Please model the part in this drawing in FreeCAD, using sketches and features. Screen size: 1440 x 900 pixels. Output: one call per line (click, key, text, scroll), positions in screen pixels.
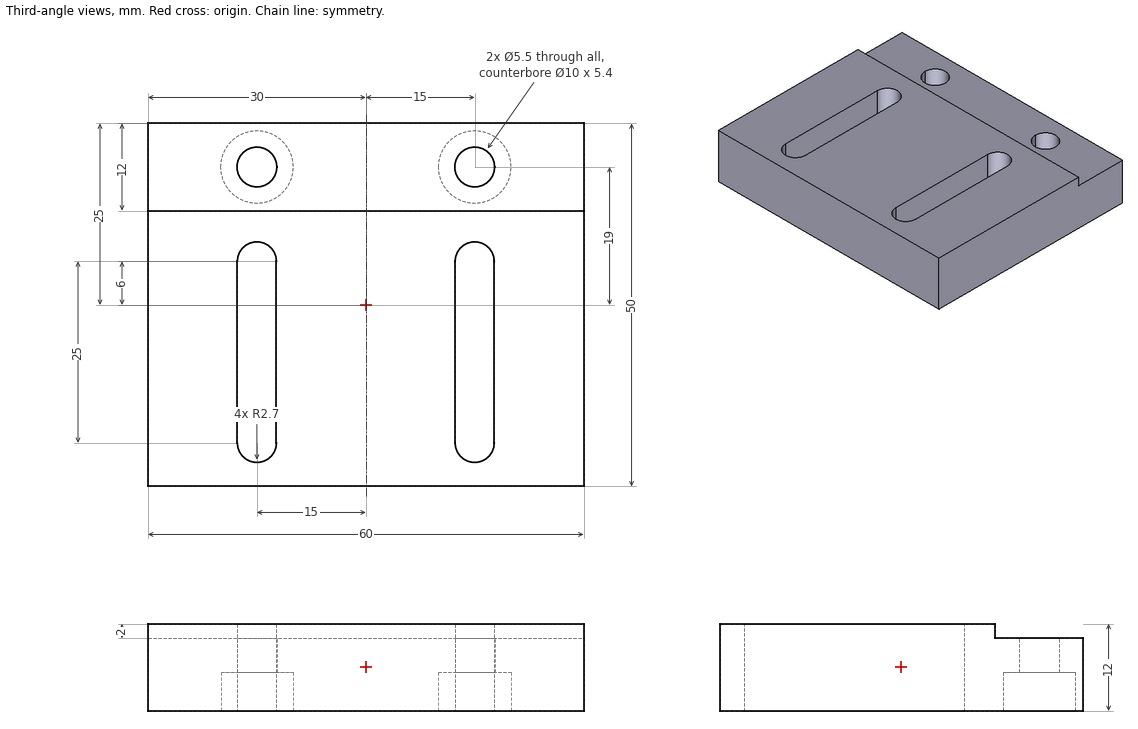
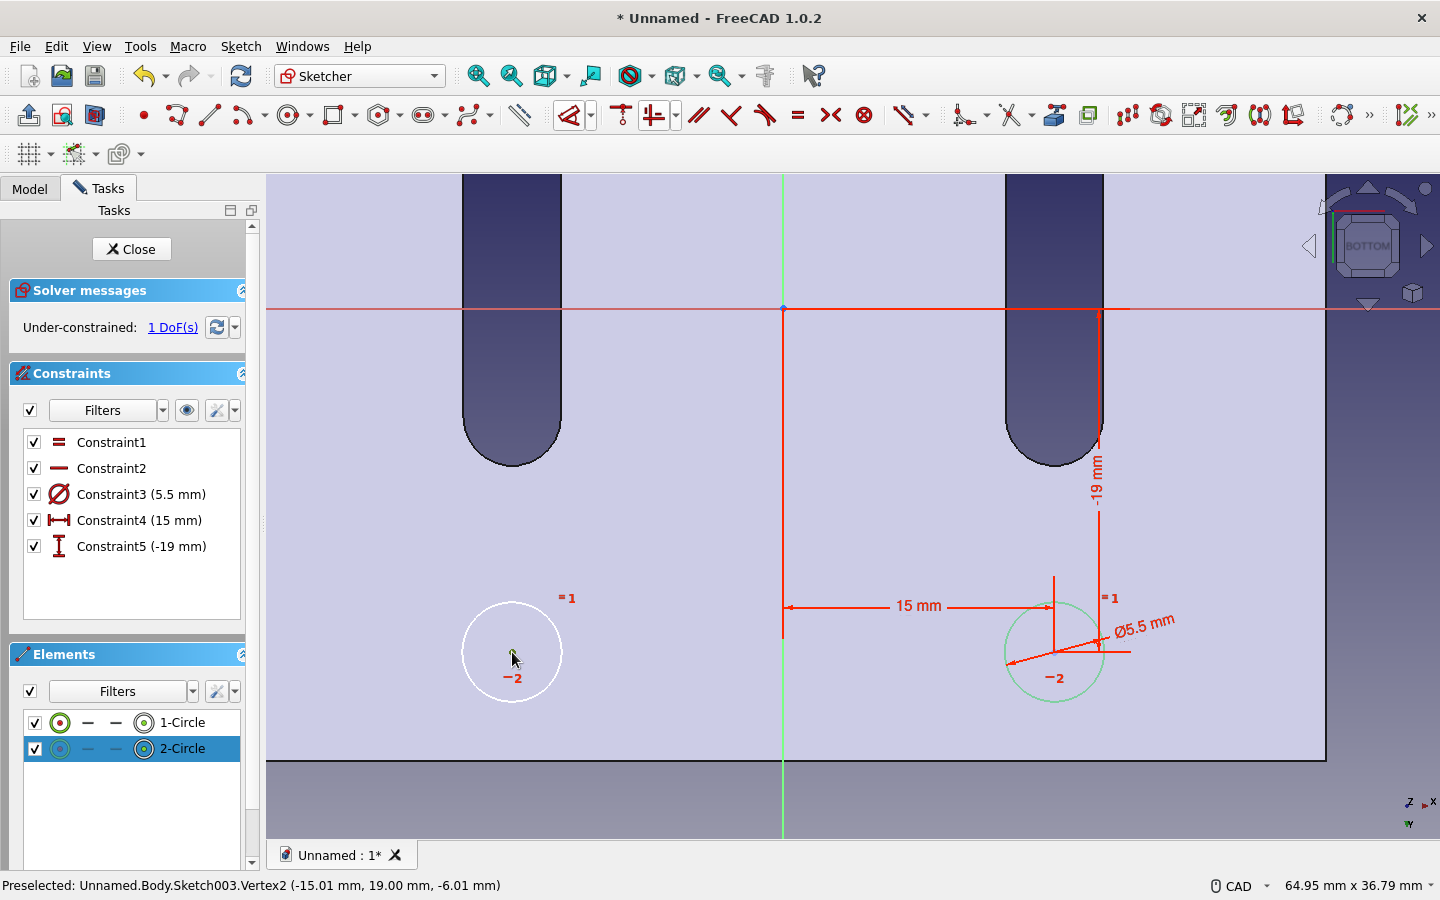
key(l)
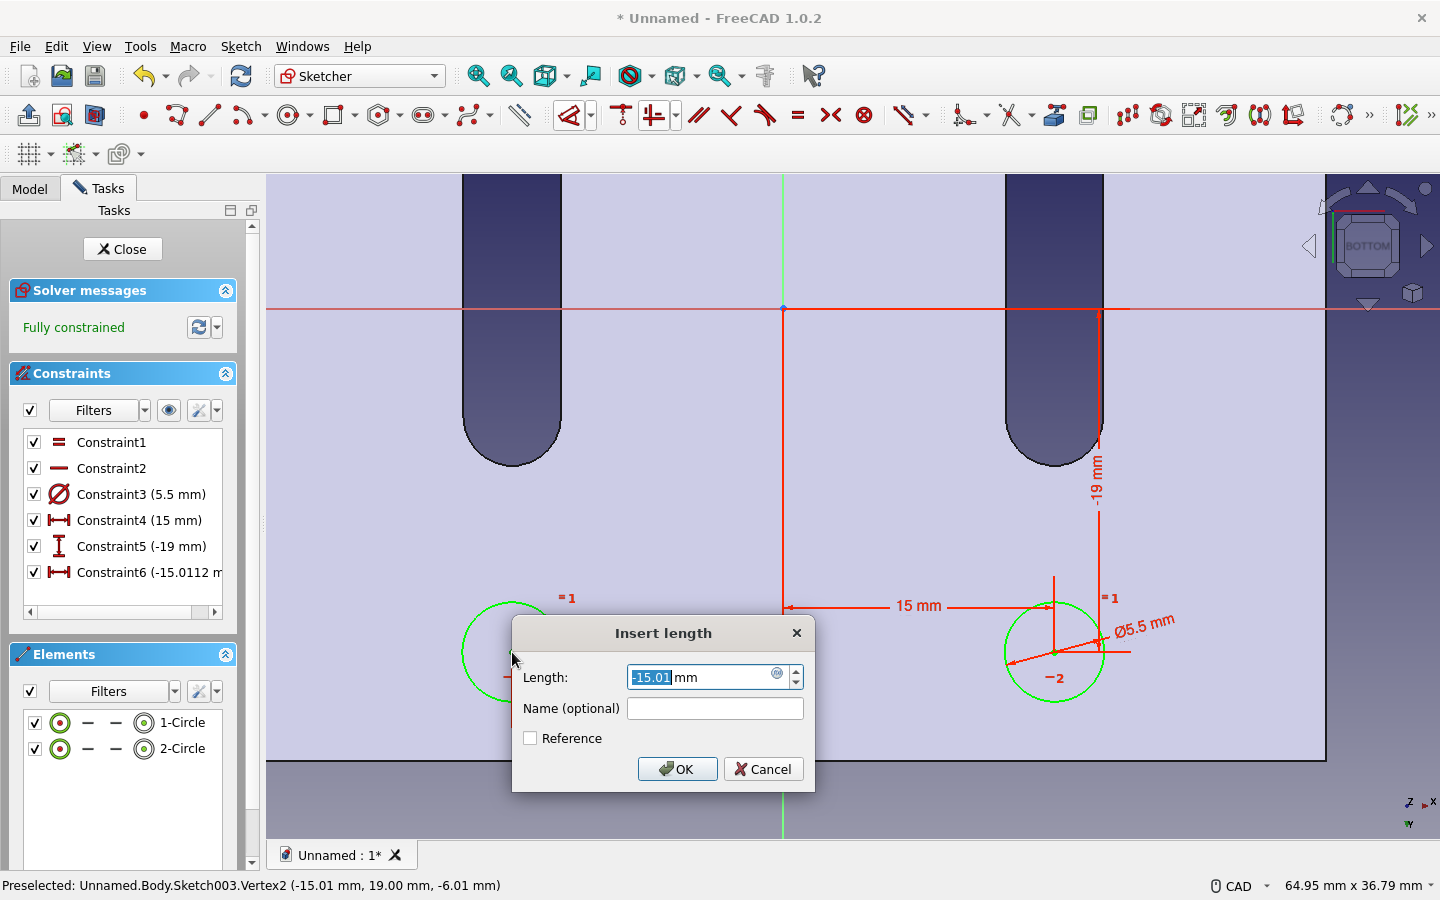
text(-15)
key(Return)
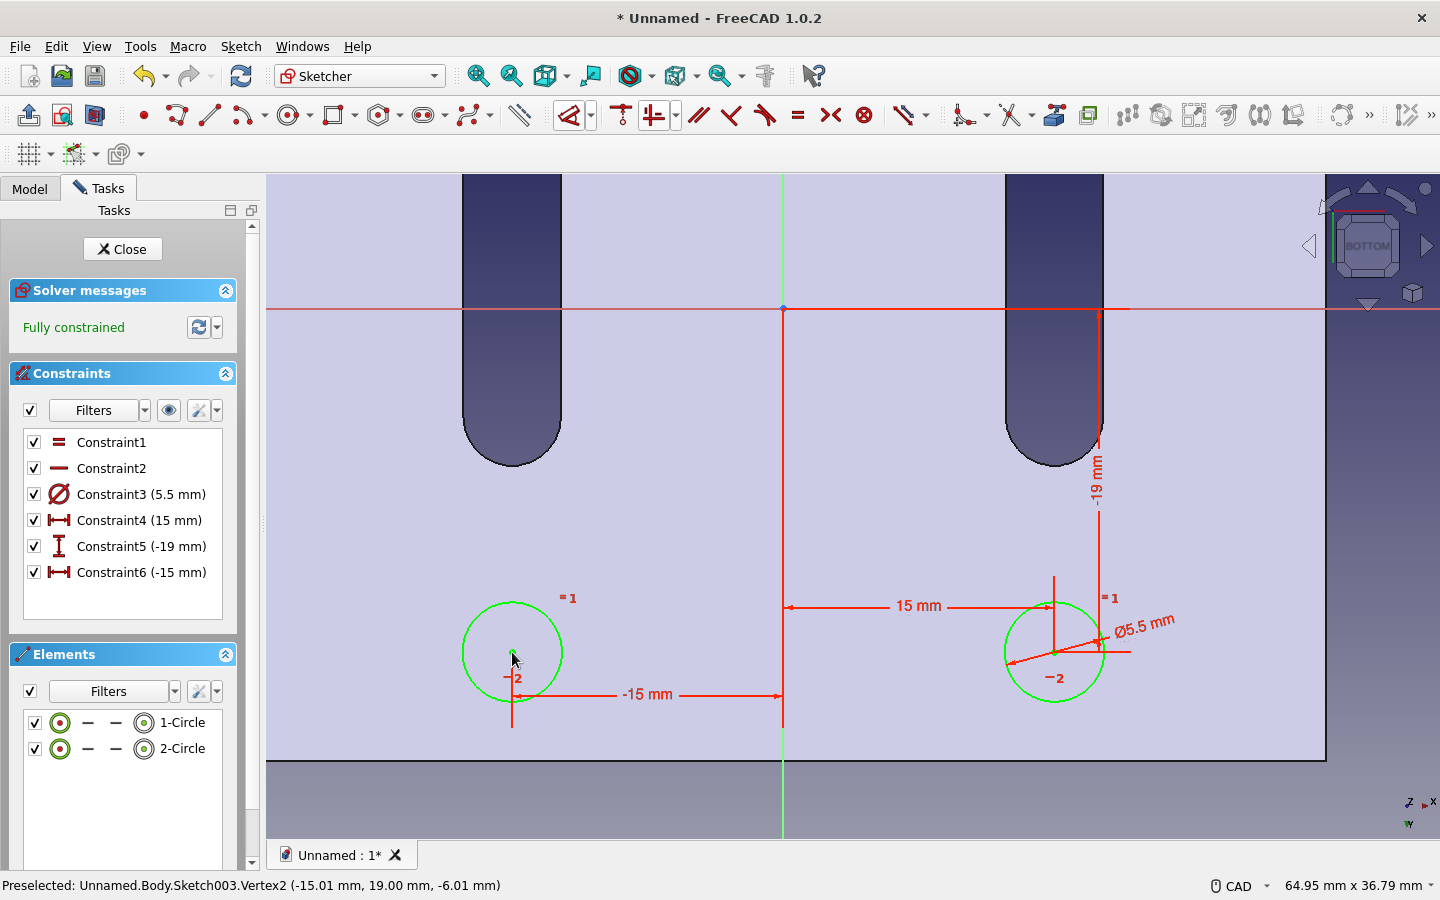
click(123, 249)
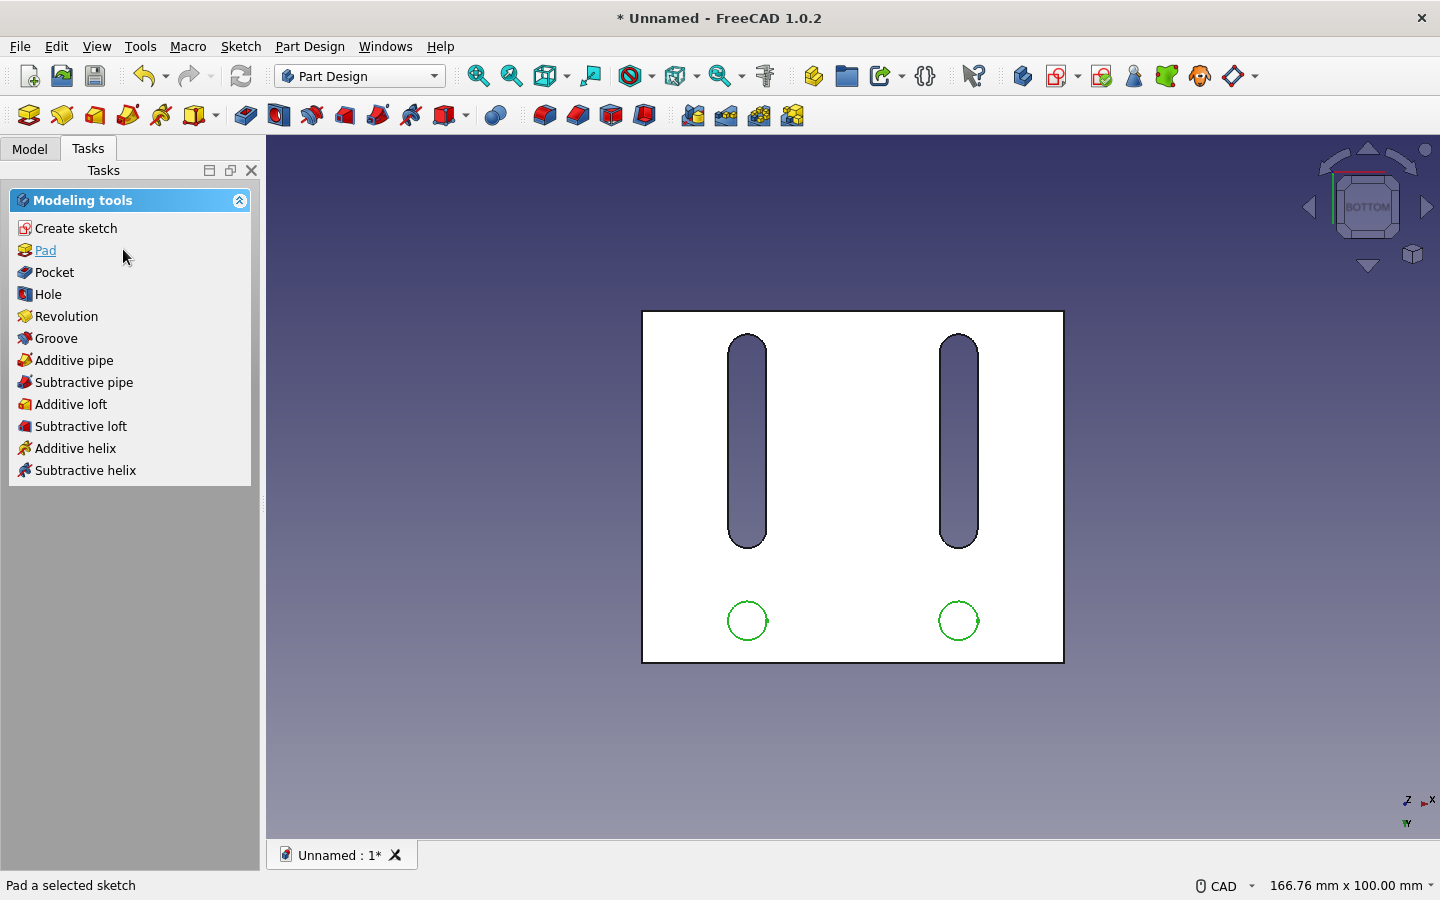
click(279, 116)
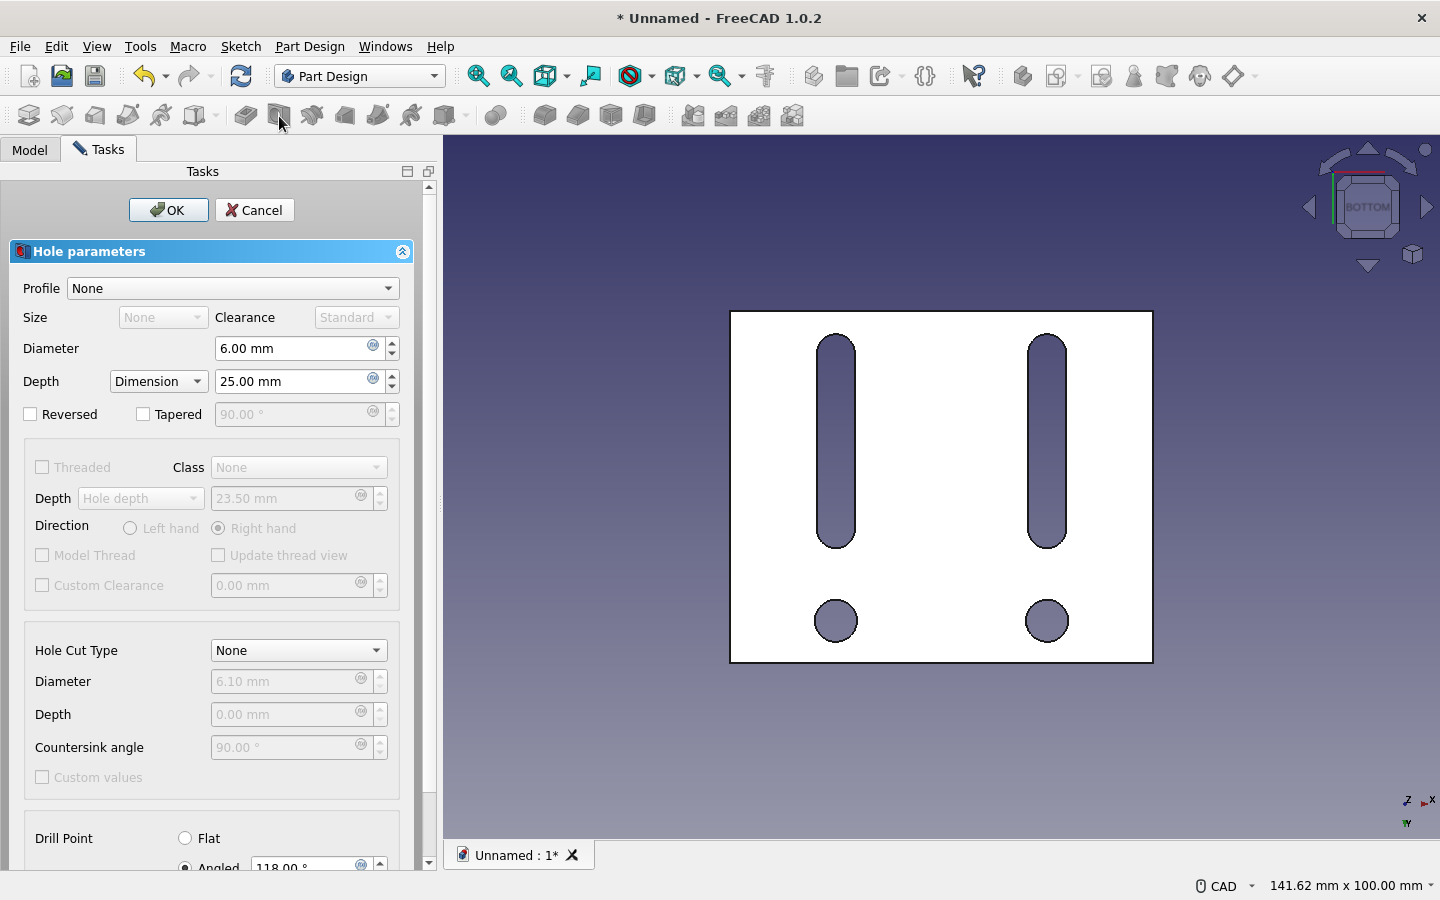
triple_click(300, 348)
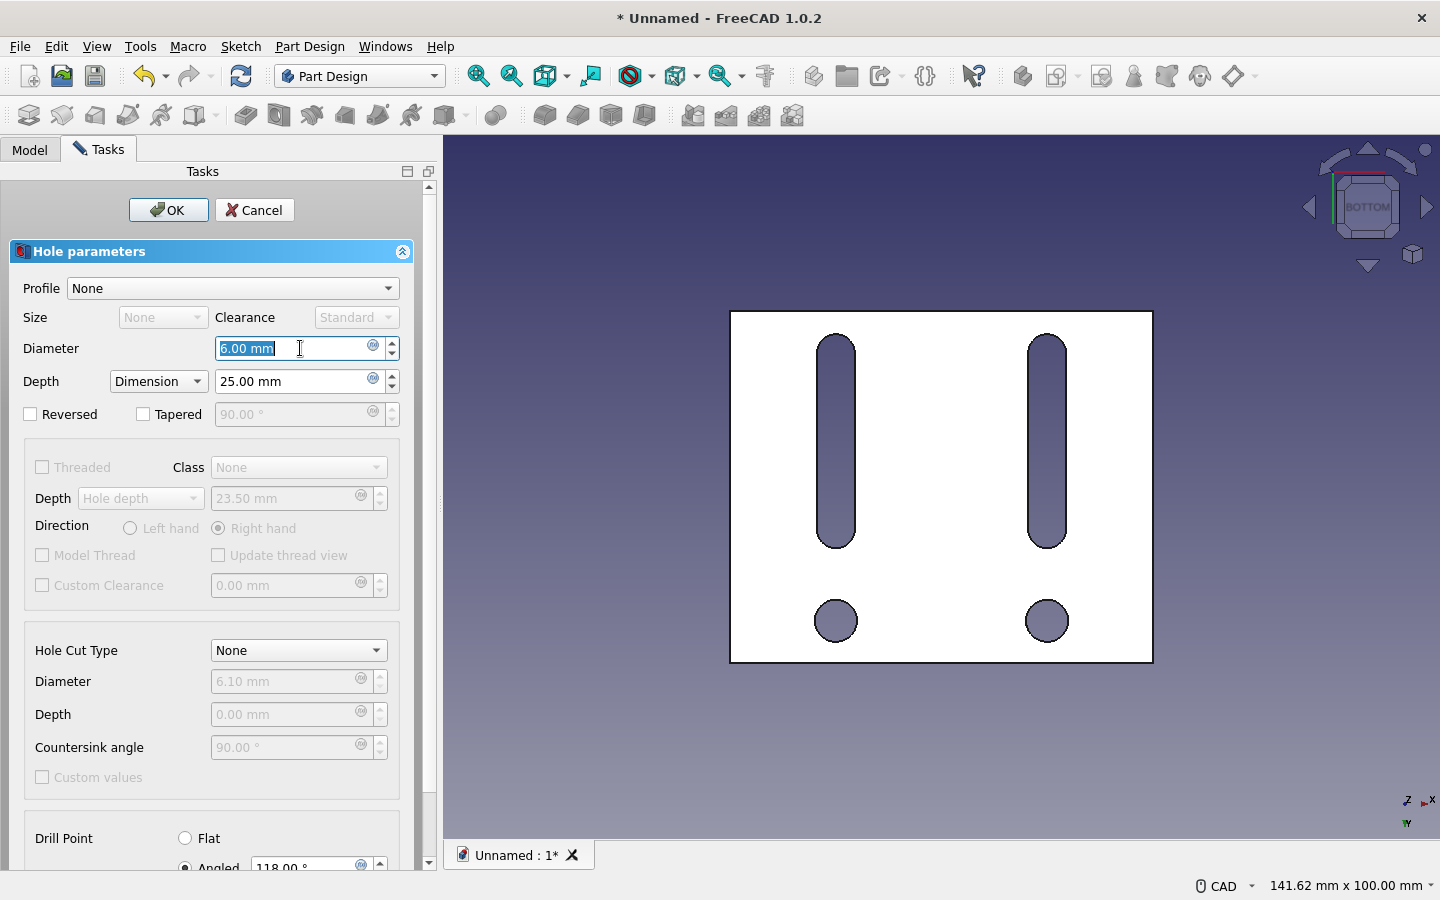
text(5.5)
key(Tab)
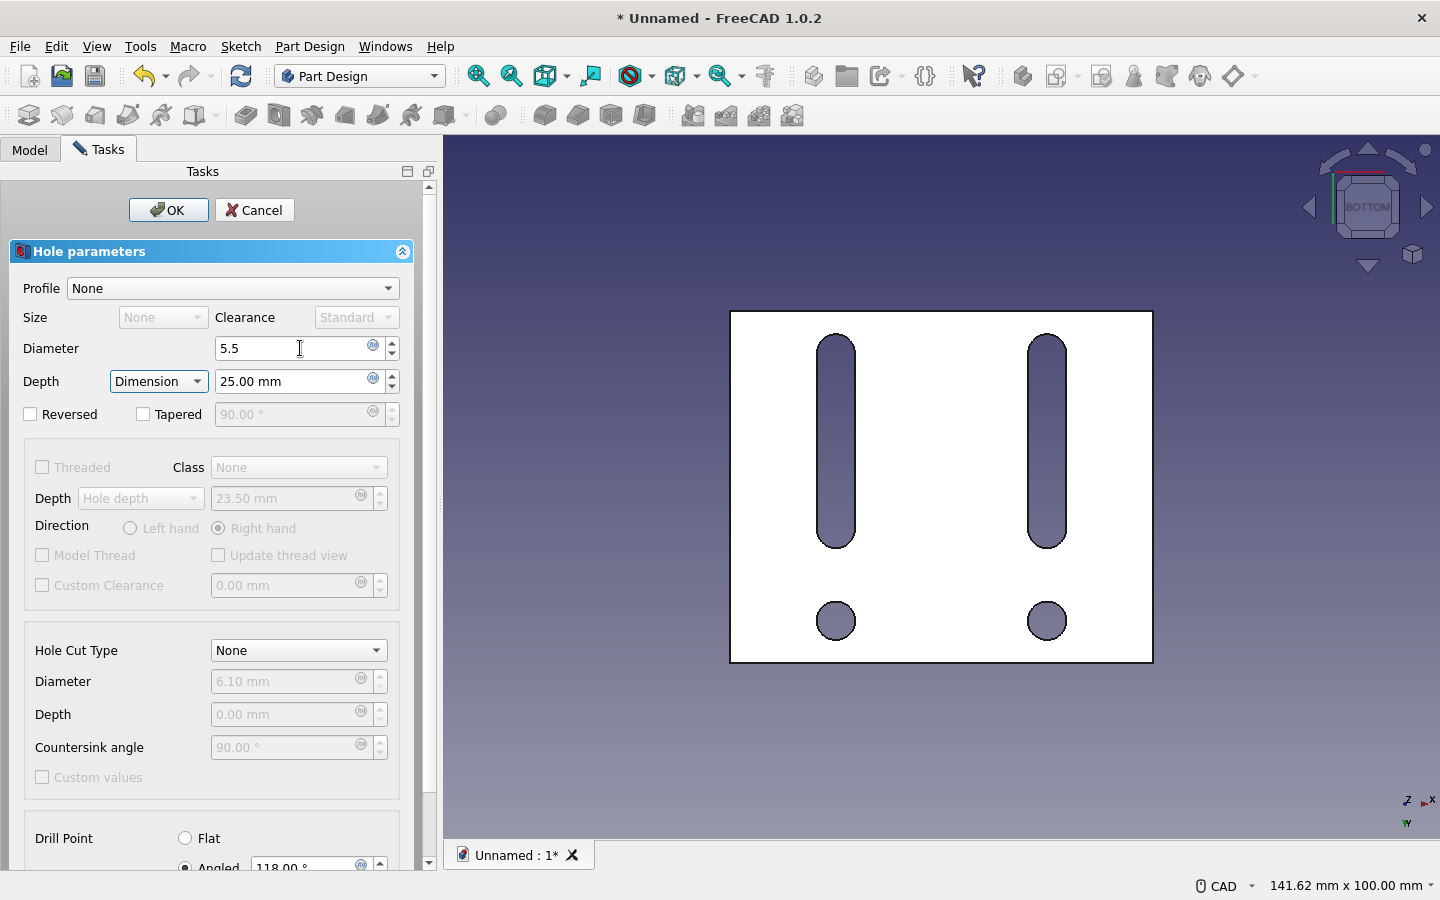
click(160, 382)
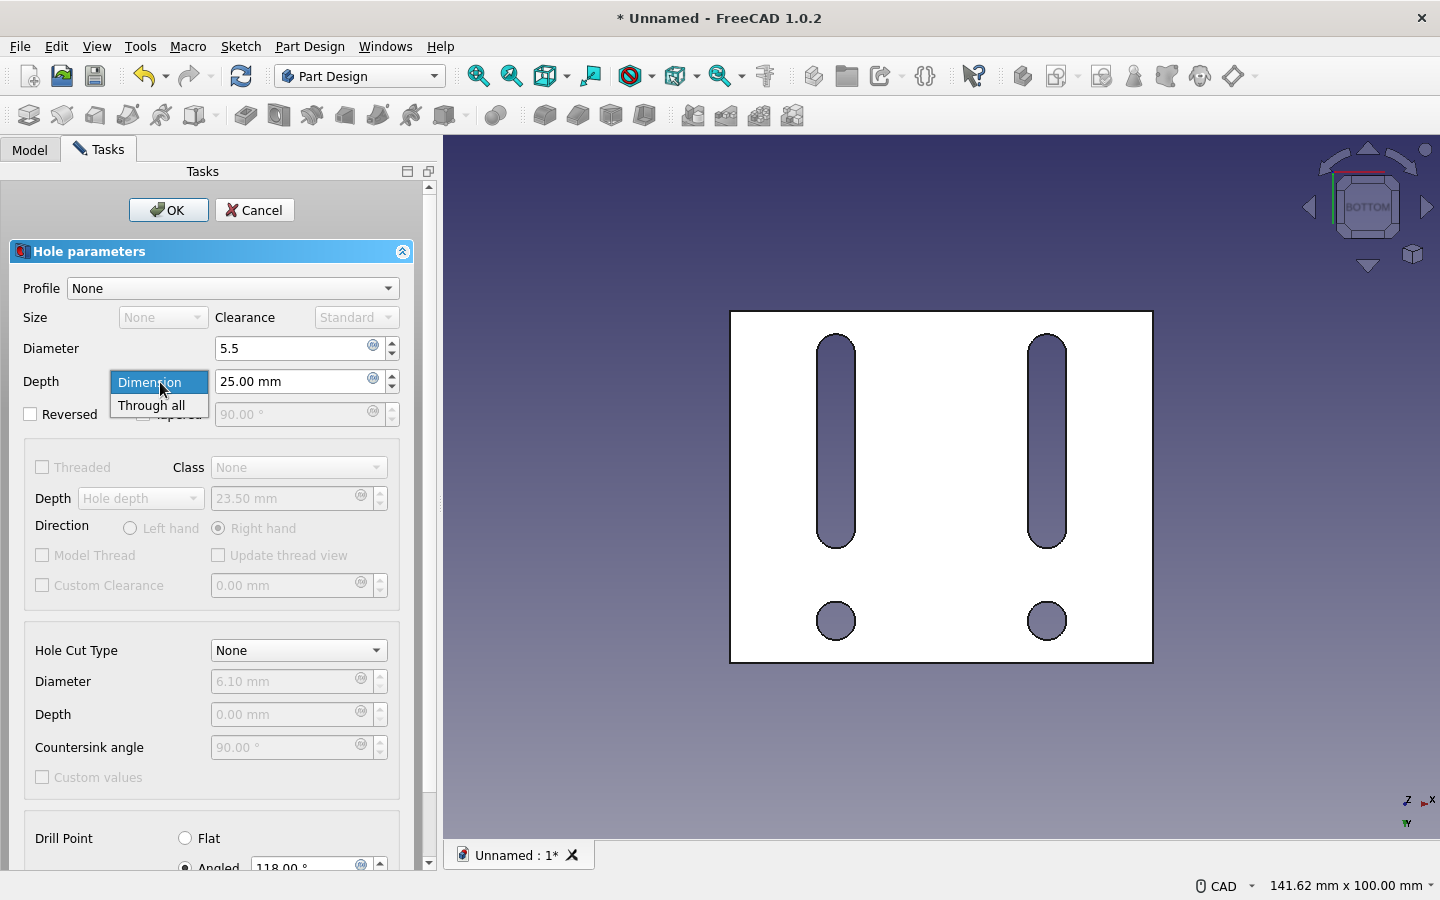
click(158, 406)